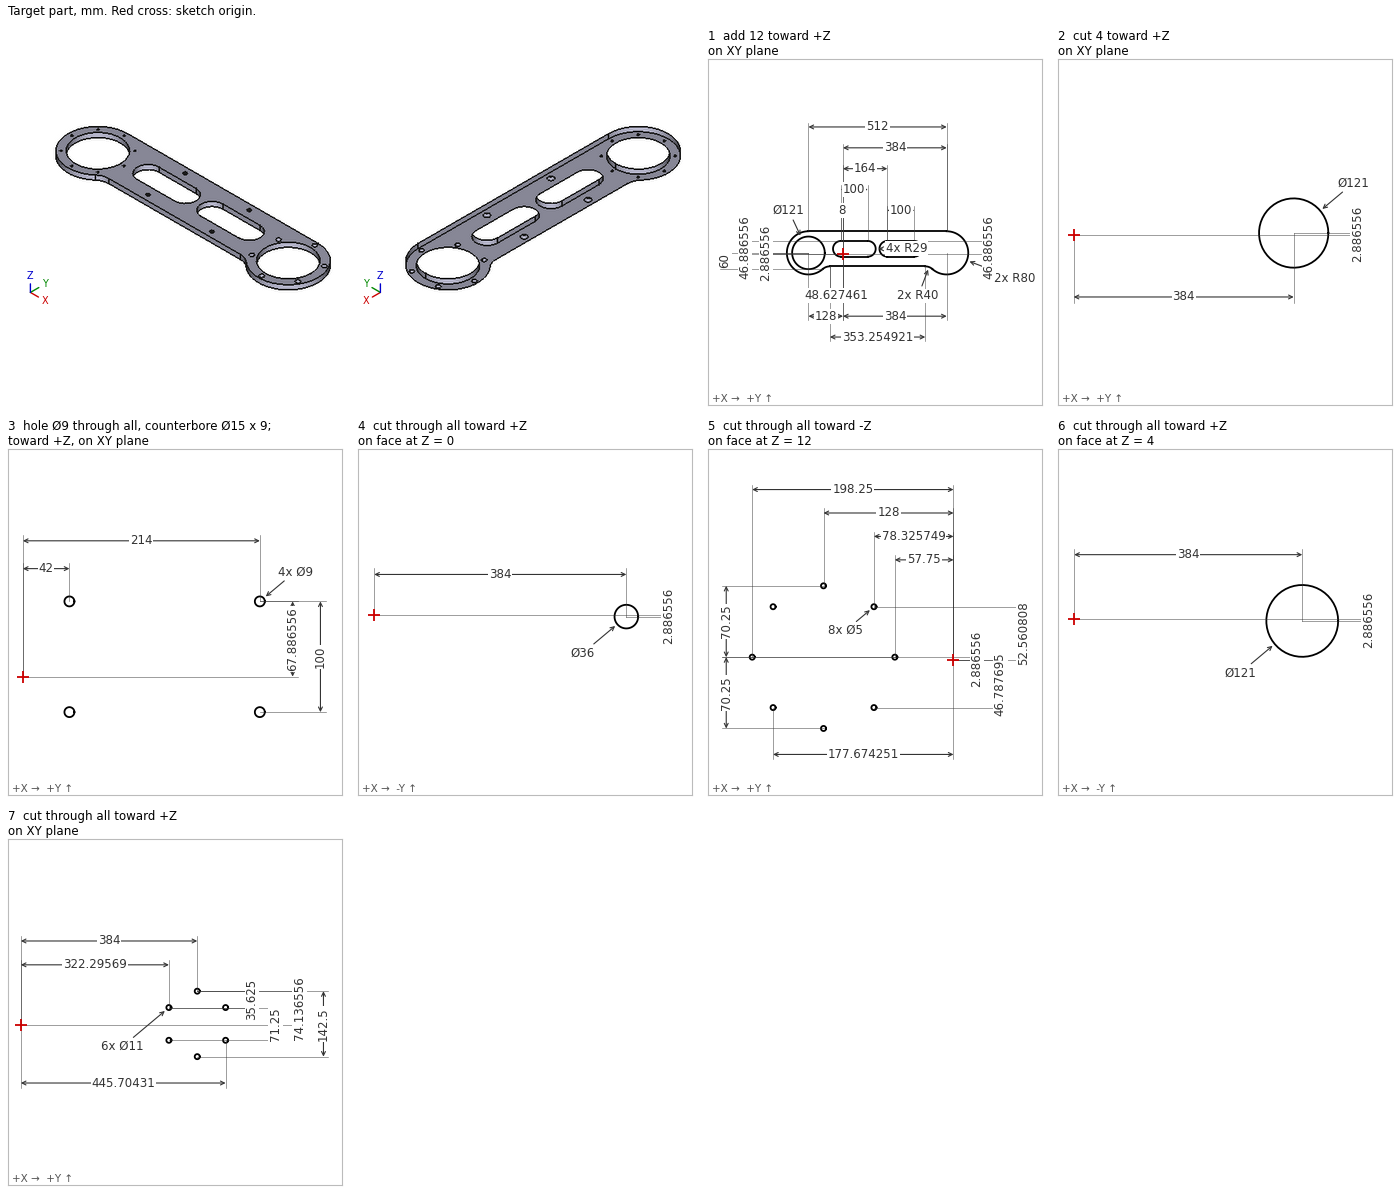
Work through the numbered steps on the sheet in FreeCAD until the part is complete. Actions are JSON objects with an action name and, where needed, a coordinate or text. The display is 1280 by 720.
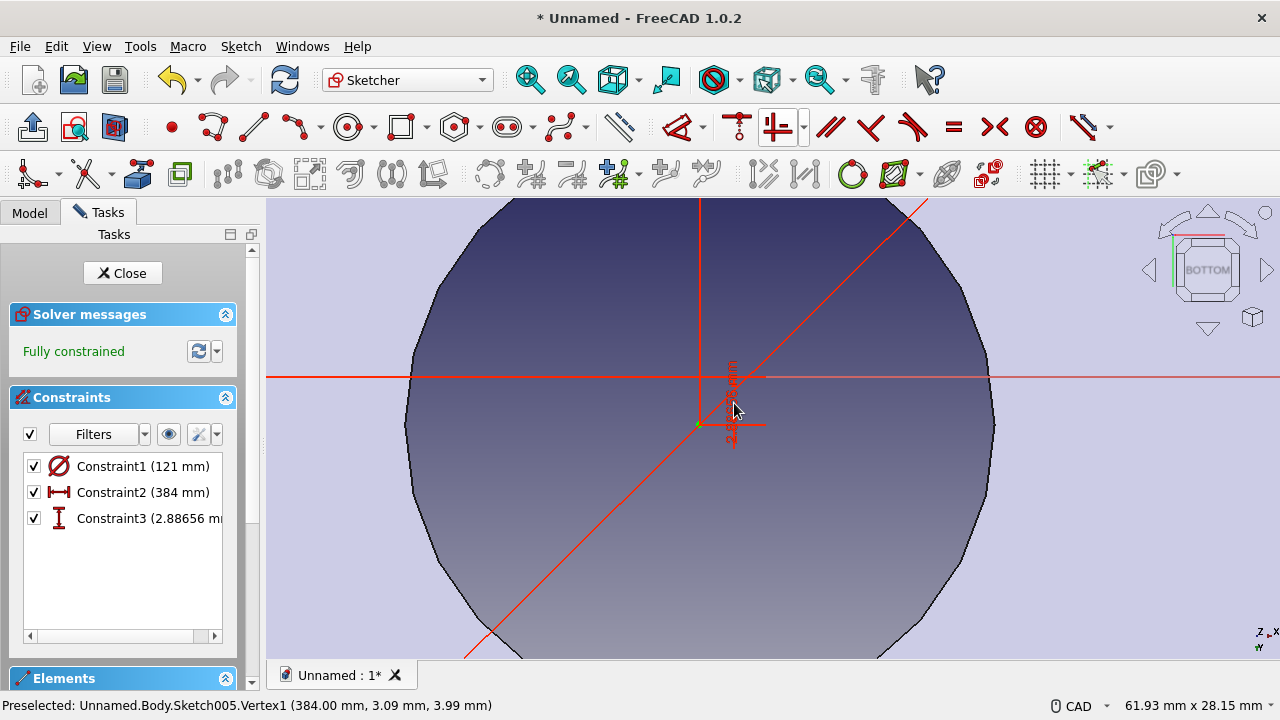
{"action": "left_click", "coordinate": [123, 273]}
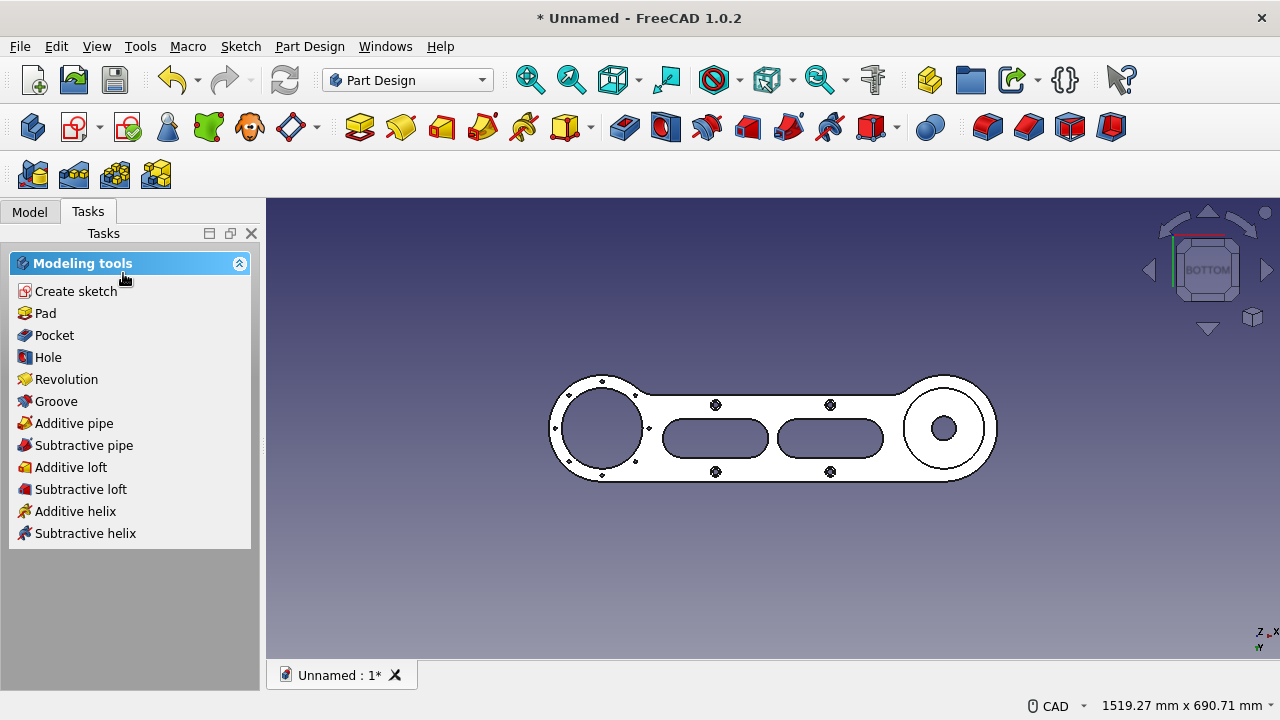
{"action": "left_click", "coordinate": [625, 128]}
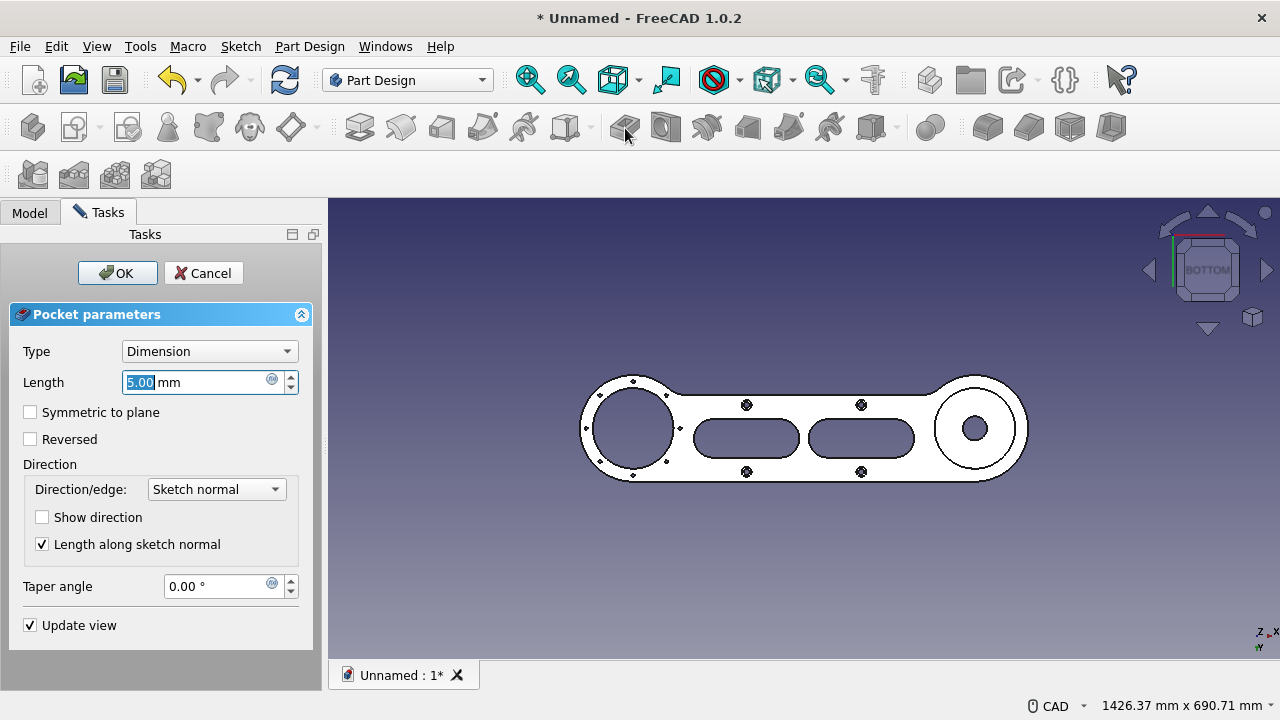
{"action": "left_click", "coordinate": [210, 352]}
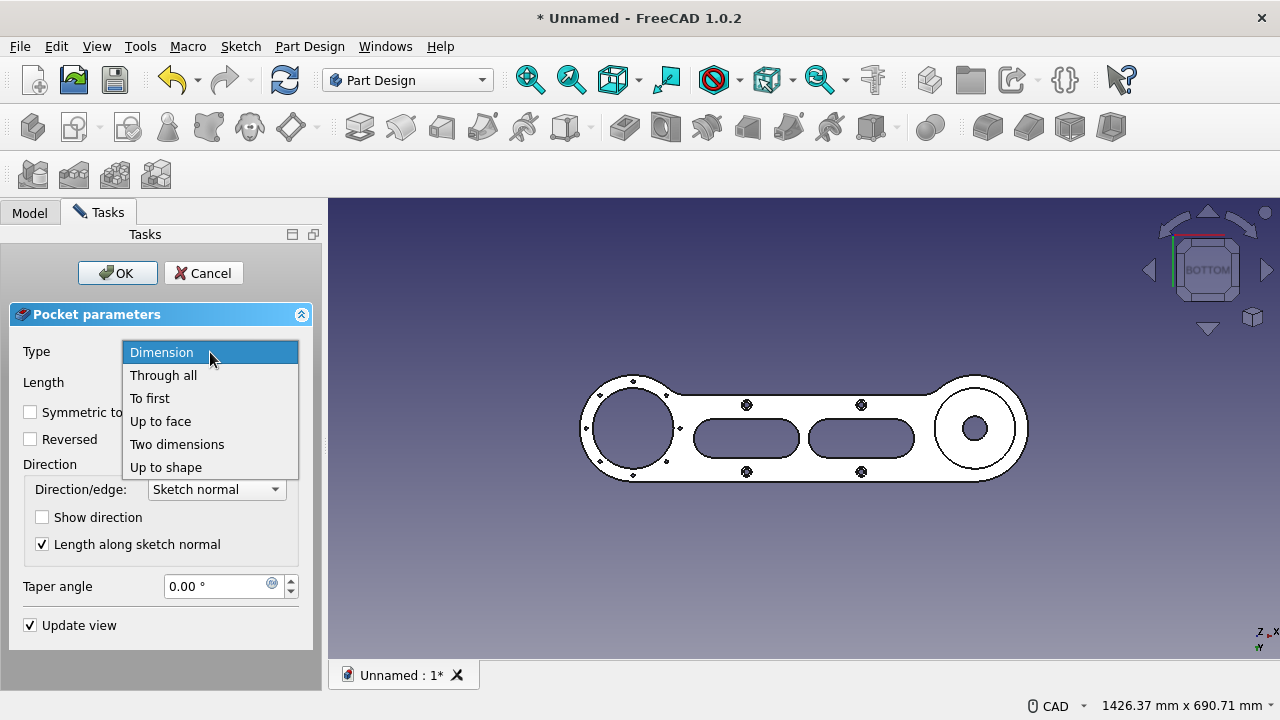
{"action": "left_click", "coordinate": [208, 376]}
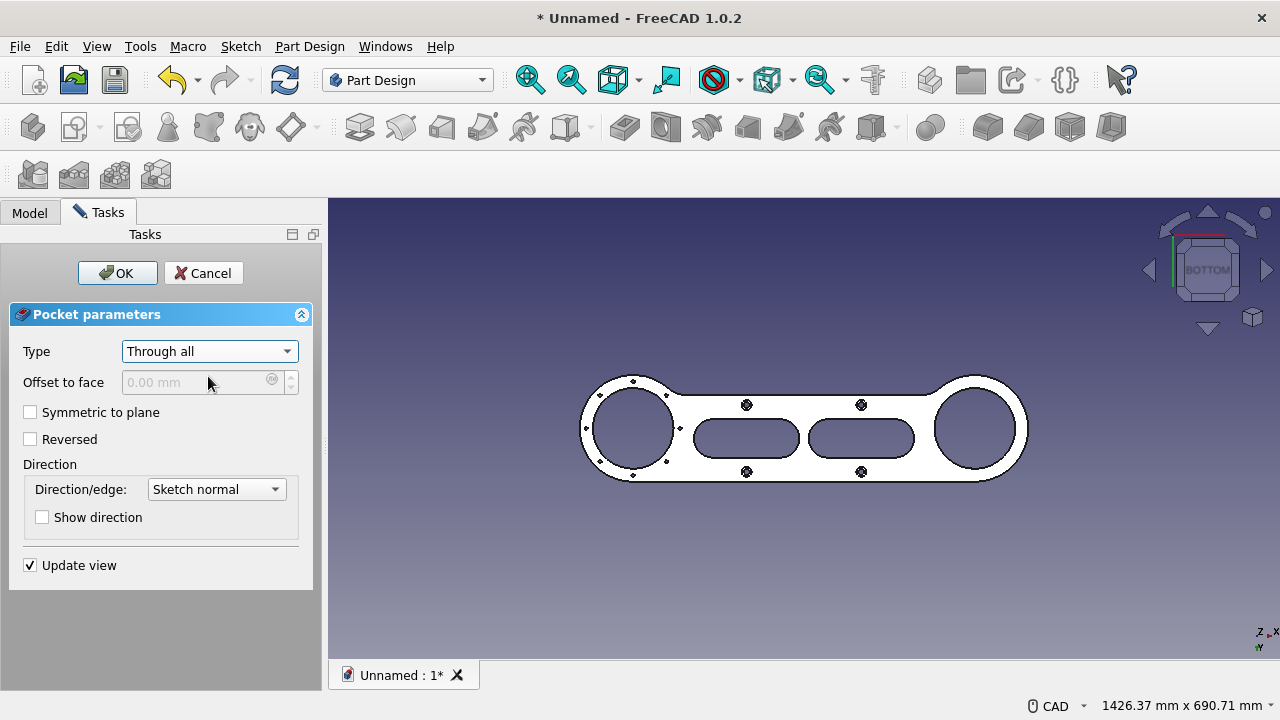
{"action": "left_click", "coordinate": [118, 273]}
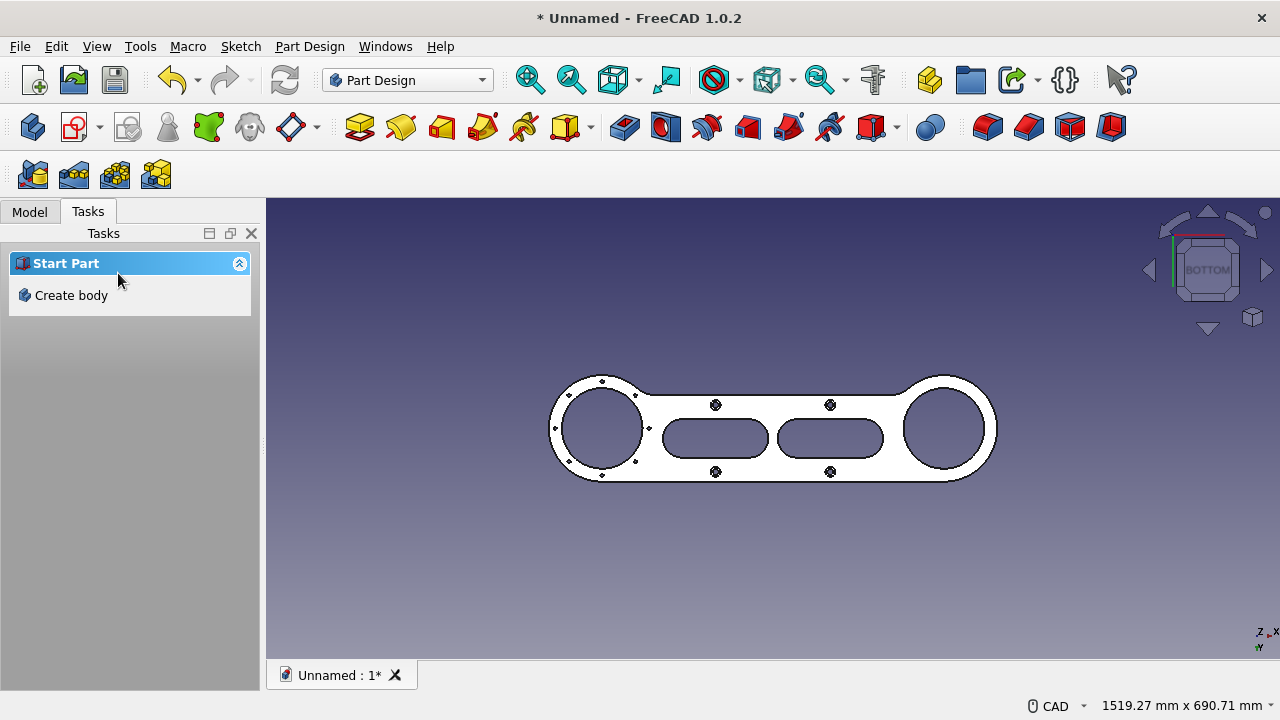
{"action": "left_click", "coordinate": [531, 80]}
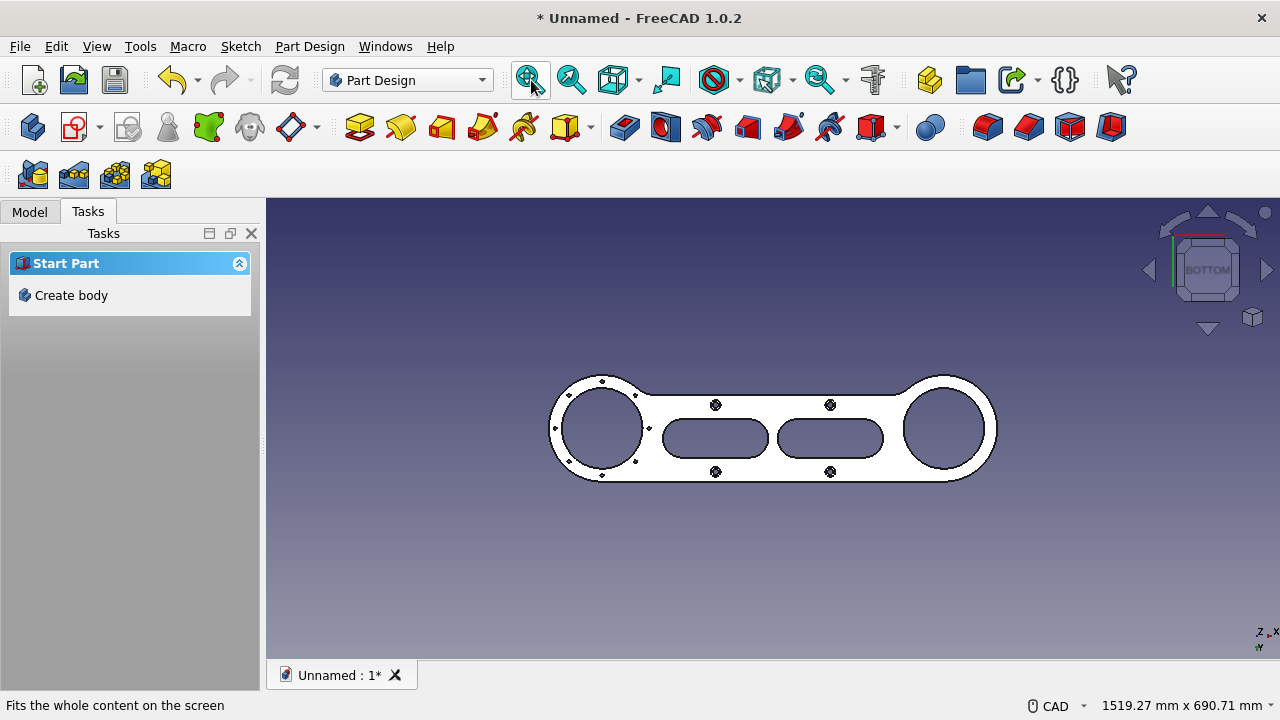
{"action": "left_click", "coordinate": [74, 128]}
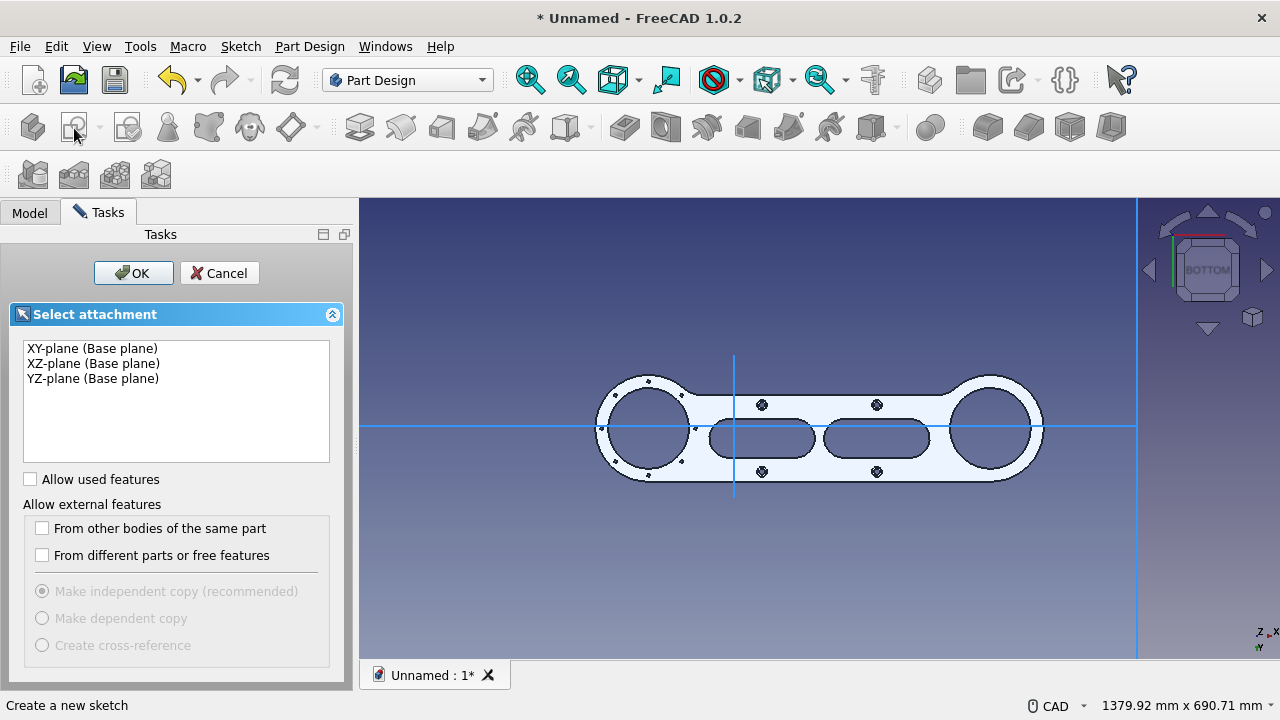
{"action": "left_click", "coordinate": [84, 348]}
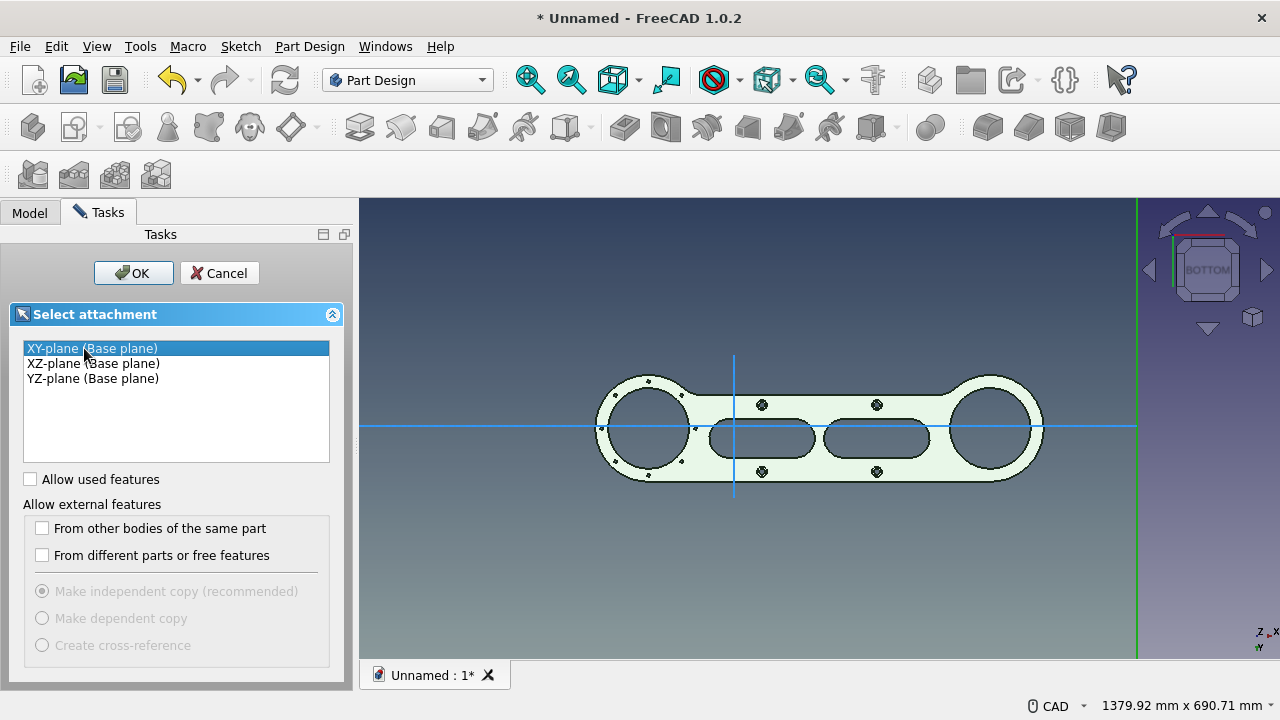
{"action": "left_click", "coordinate": [134, 273]}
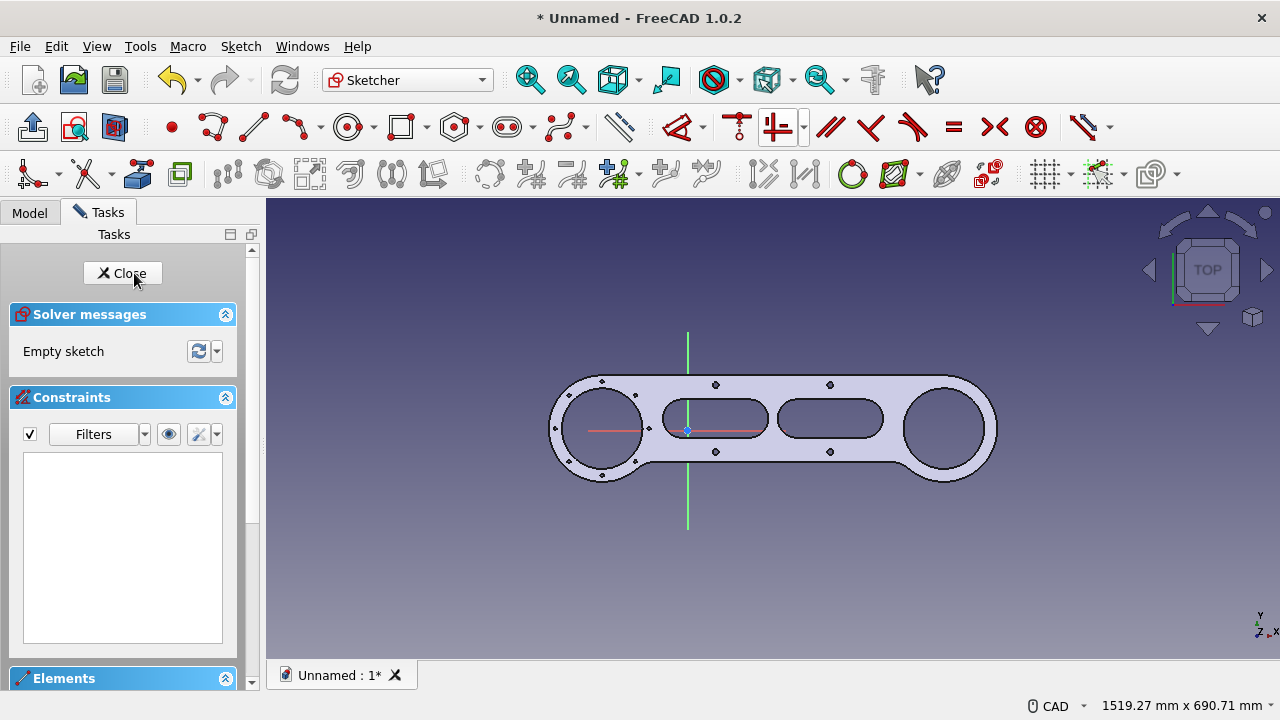
{"action": "left_click", "coordinate": [115, 128]}